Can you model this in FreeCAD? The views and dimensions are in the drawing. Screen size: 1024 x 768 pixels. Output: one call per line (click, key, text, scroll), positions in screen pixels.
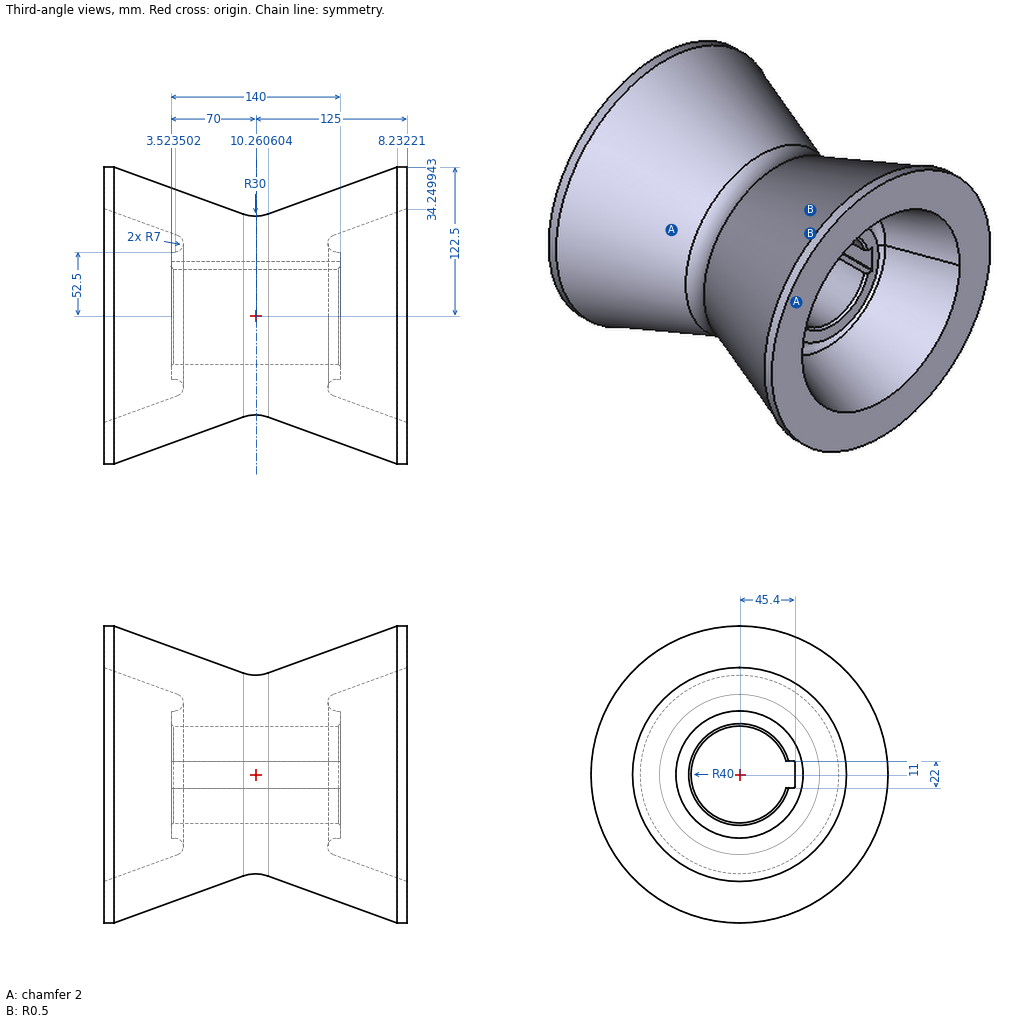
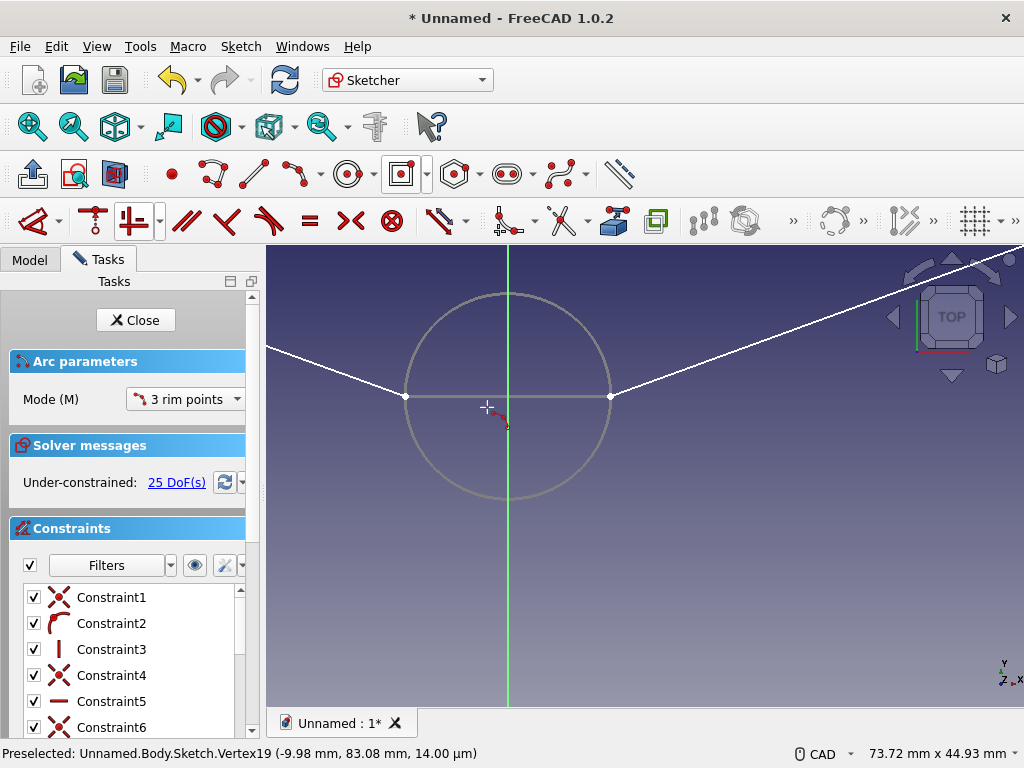
click(486, 408)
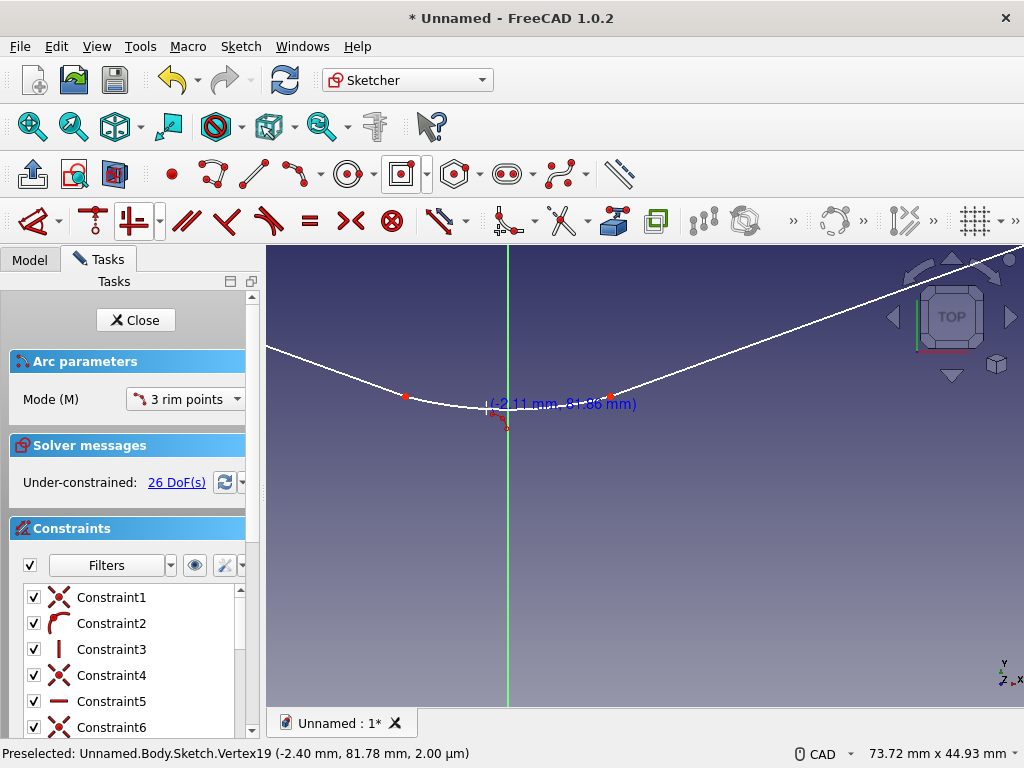
scroll(590, 447, down, 9)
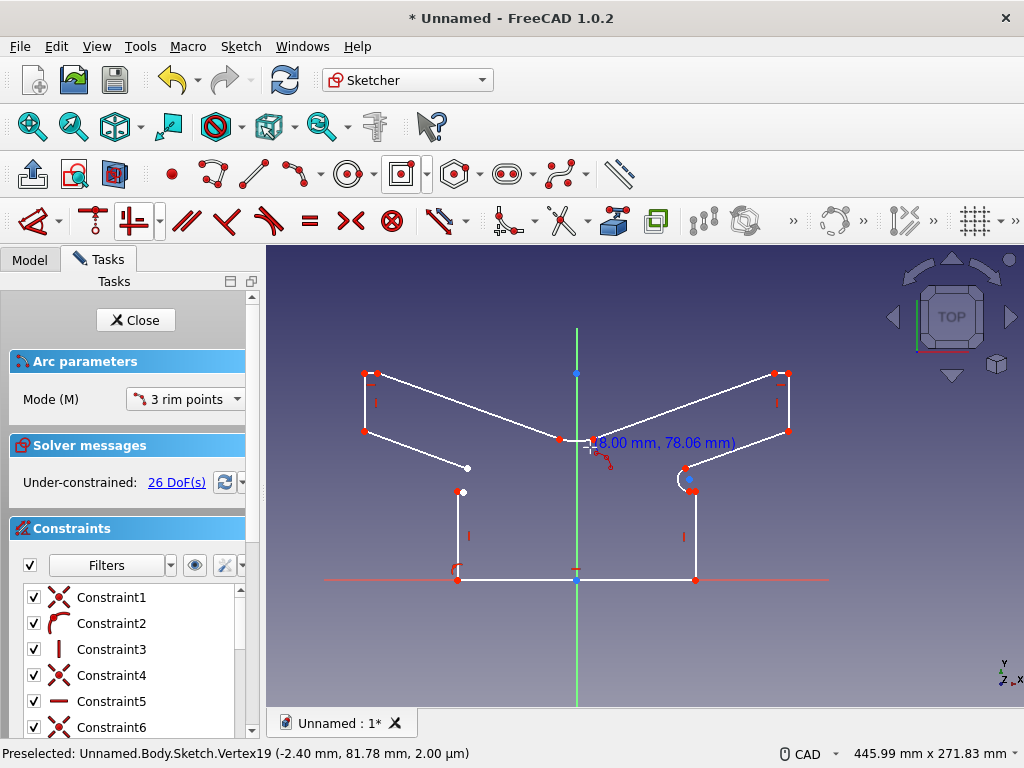
click(468, 469)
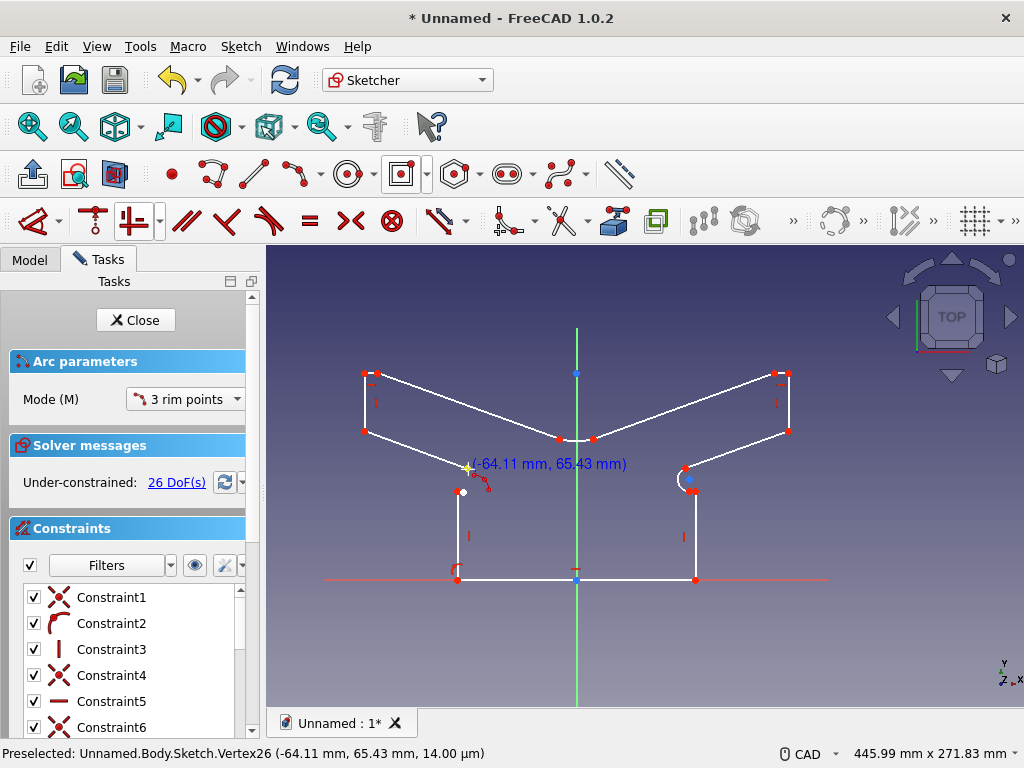
scroll(464, 491, up, 9)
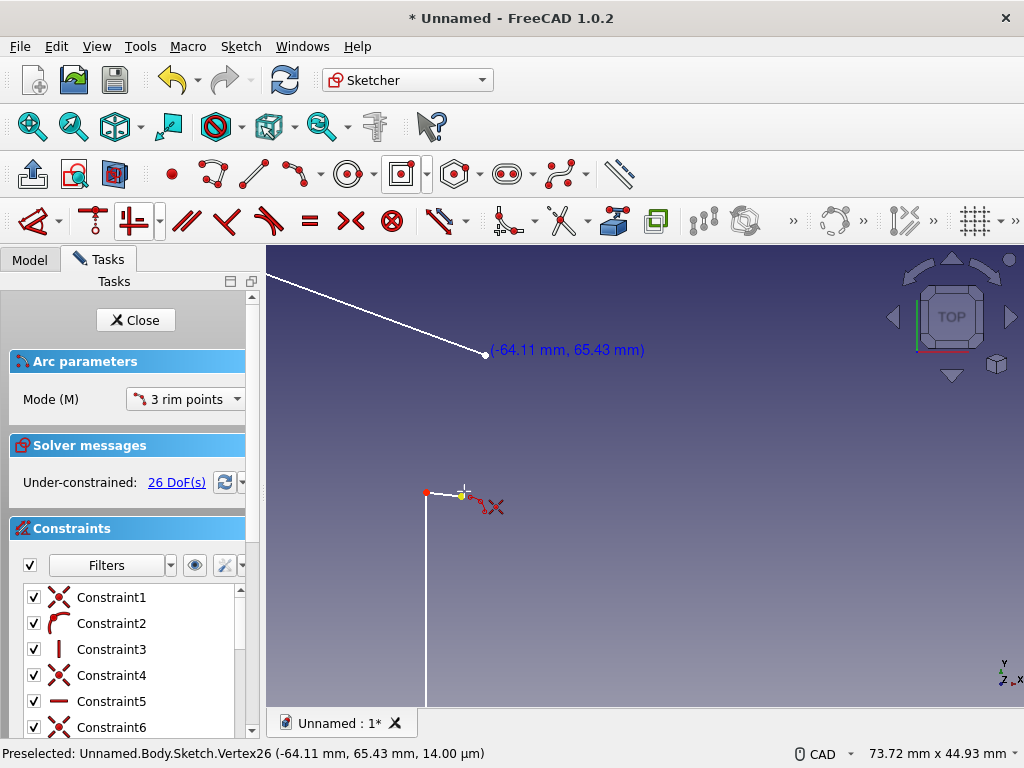
click(461, 497)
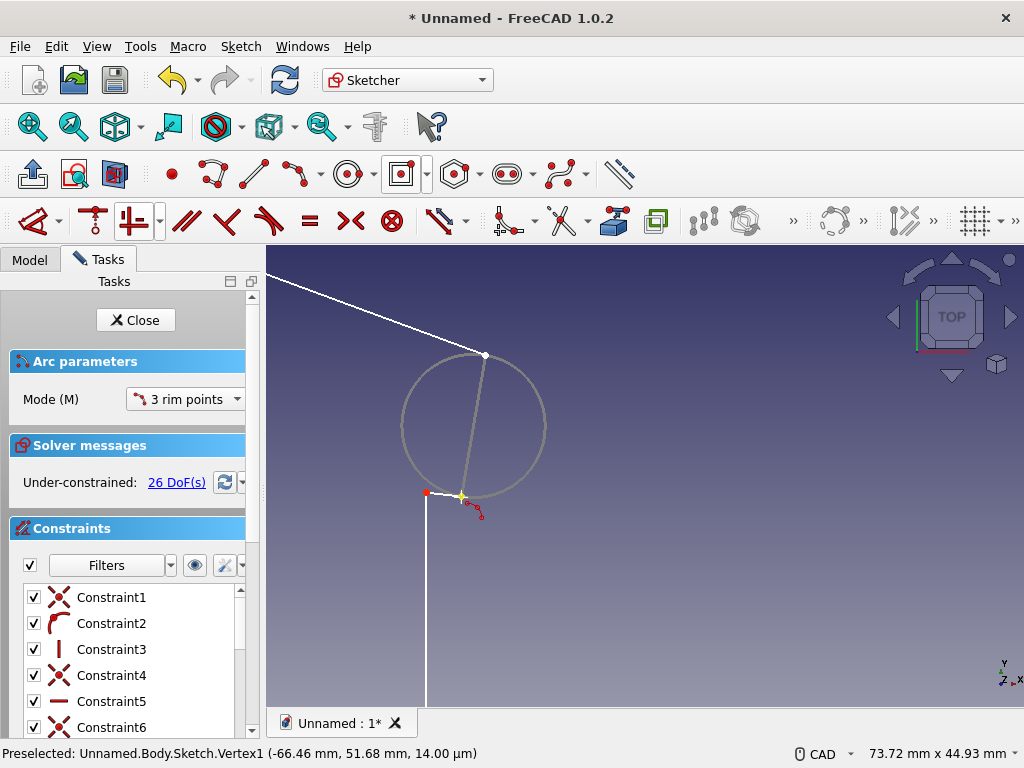
scroll(464, 491, down, 9)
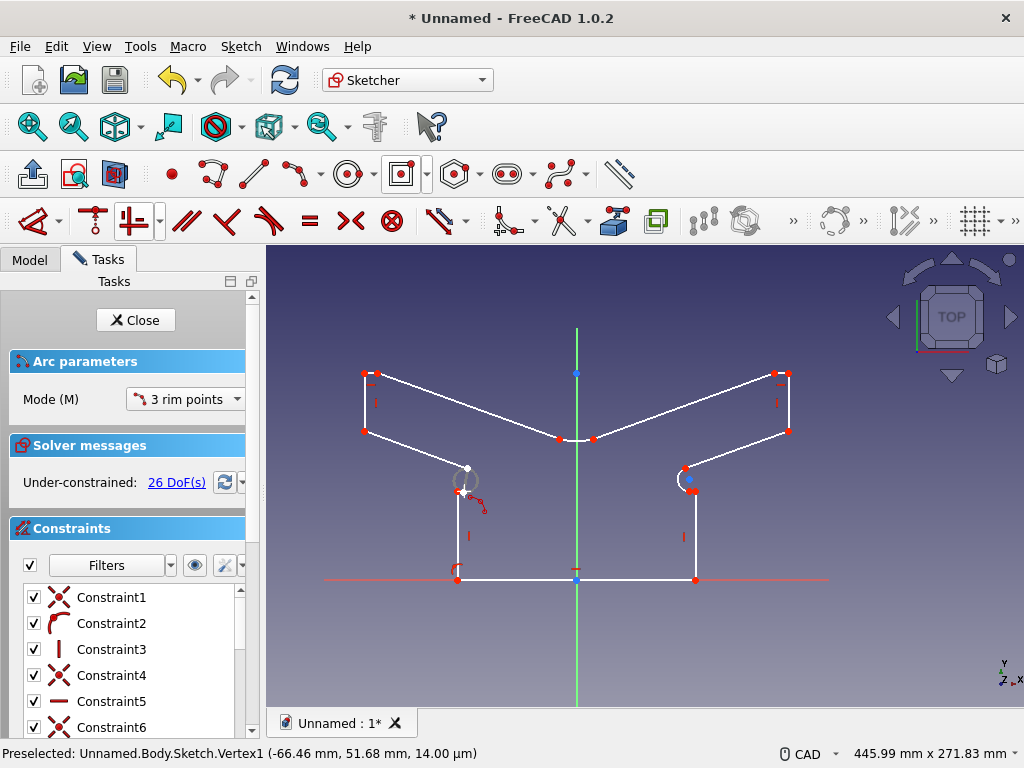
scroll(475, 481, up, 3)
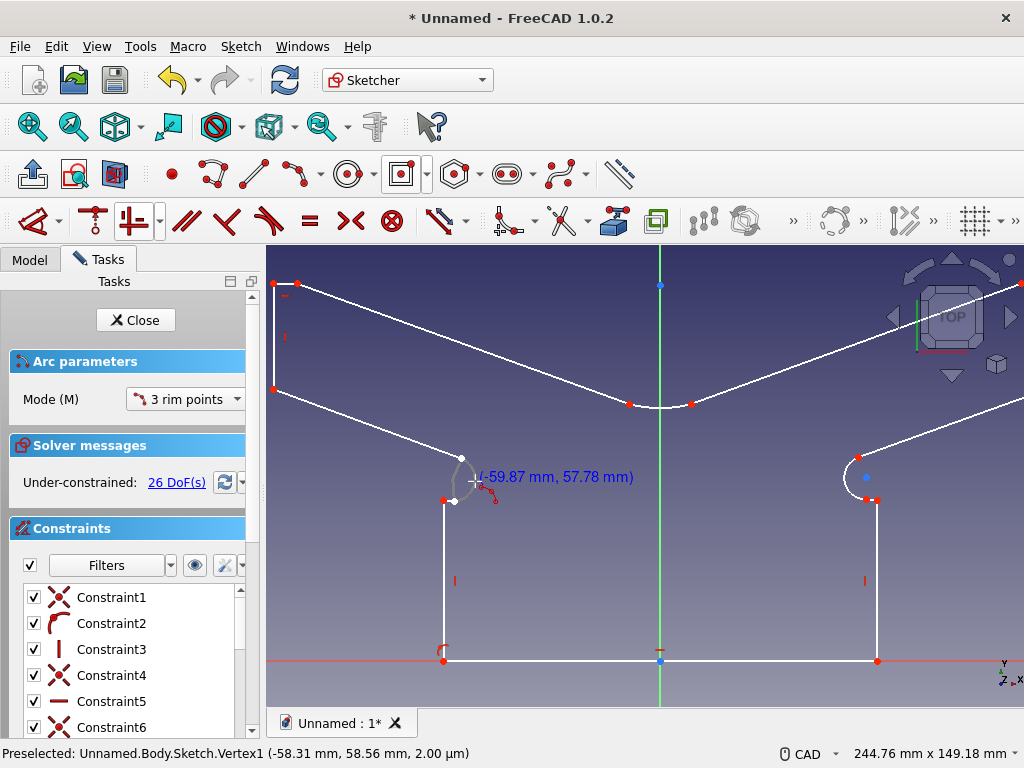
click(476, 481)
key(Escape)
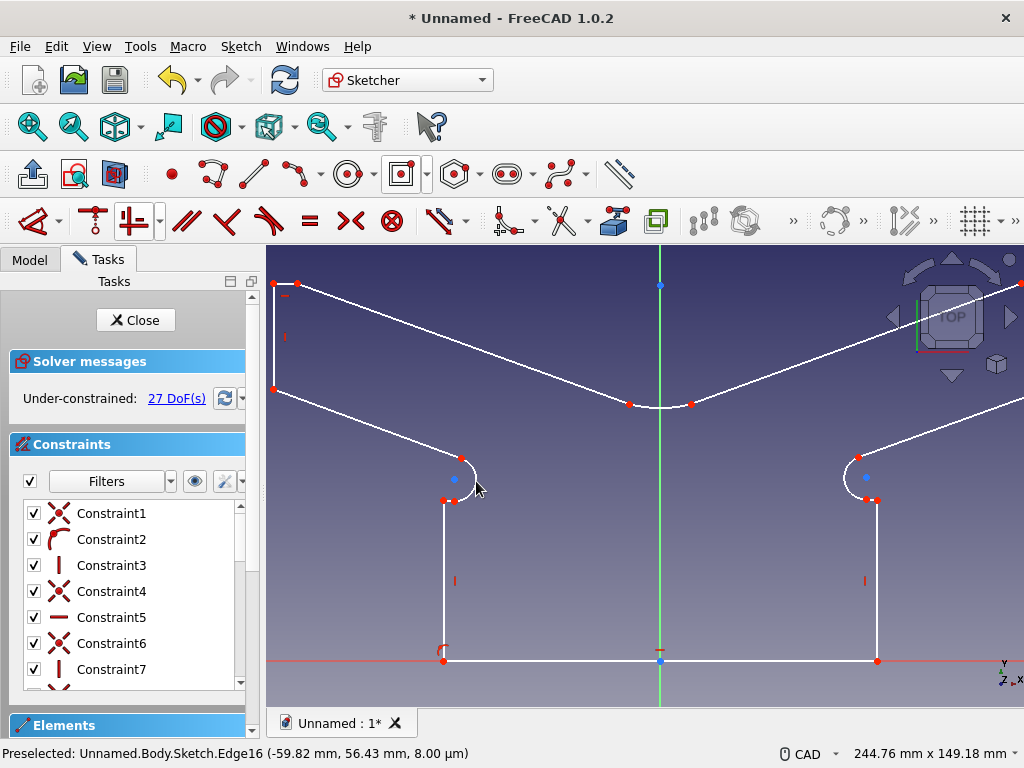
scroll(449, 501, up, 5)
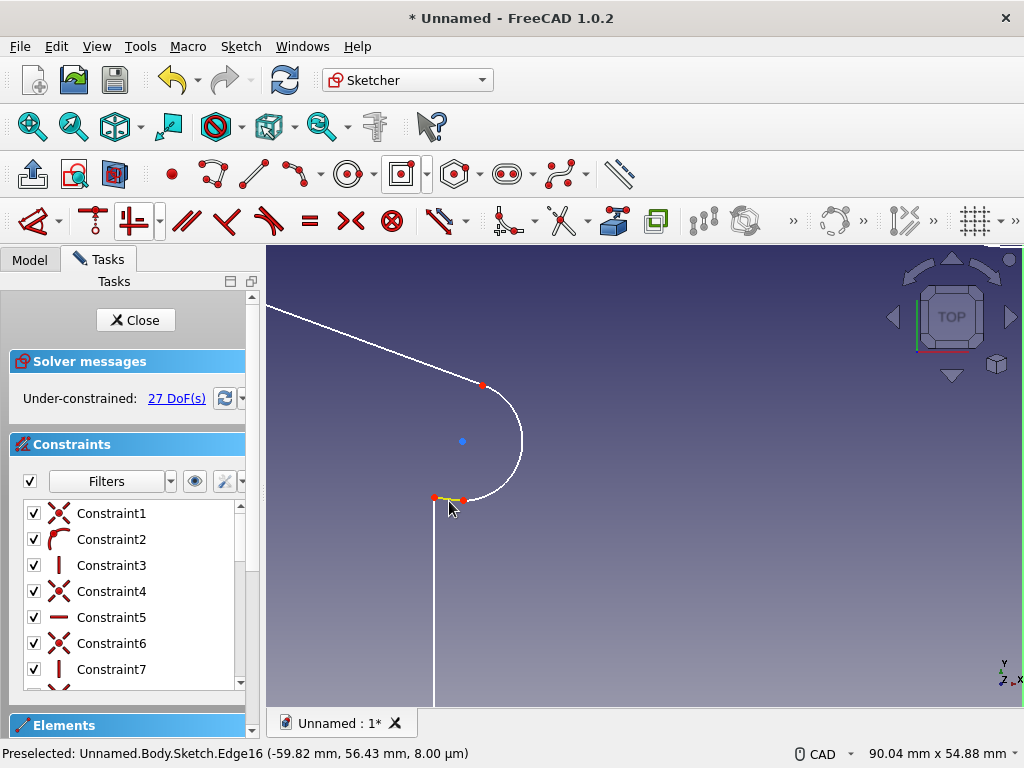
click(449, 499)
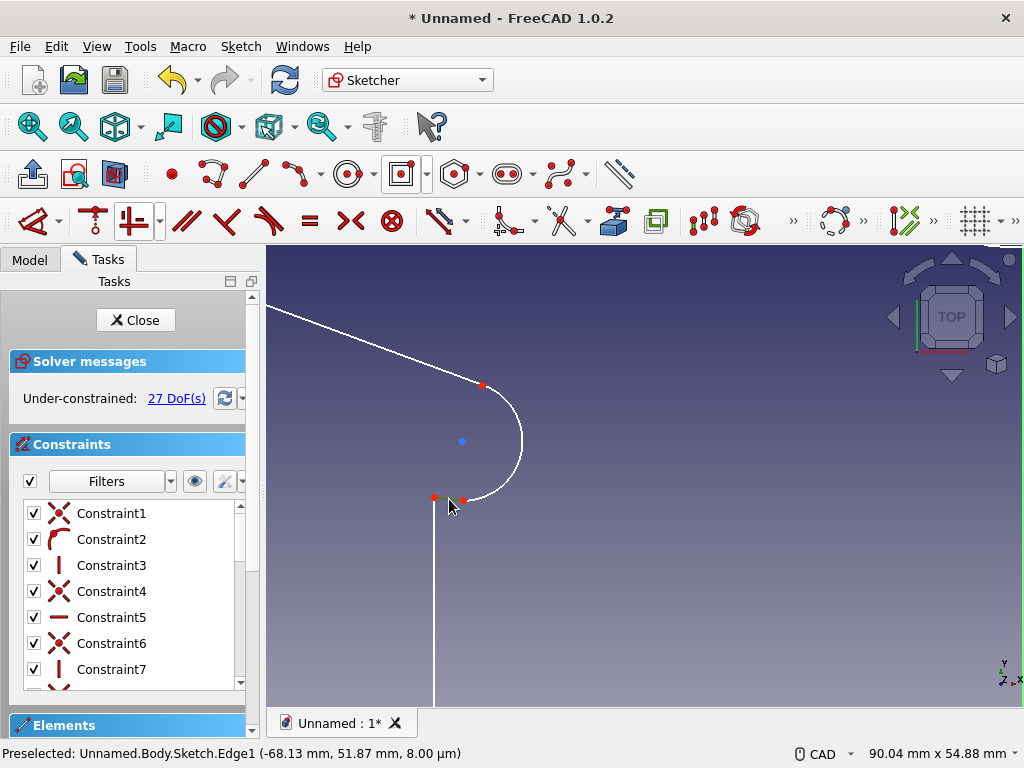
scroll(464, 490, down, 8)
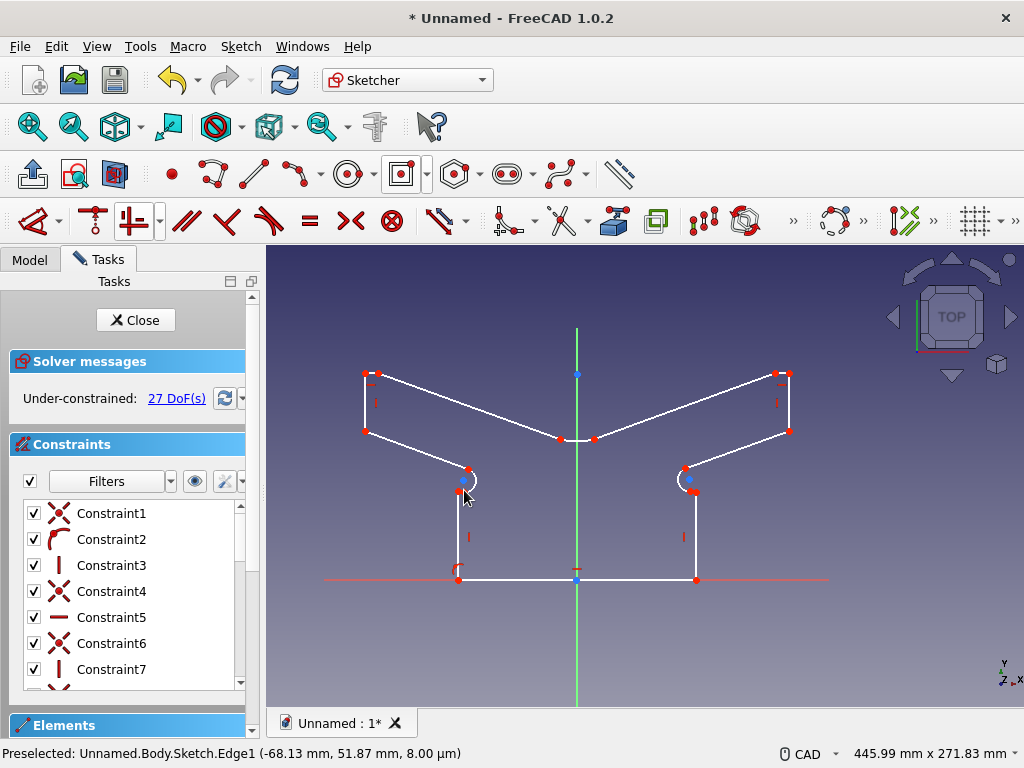
scroll(473, 489, up, 2)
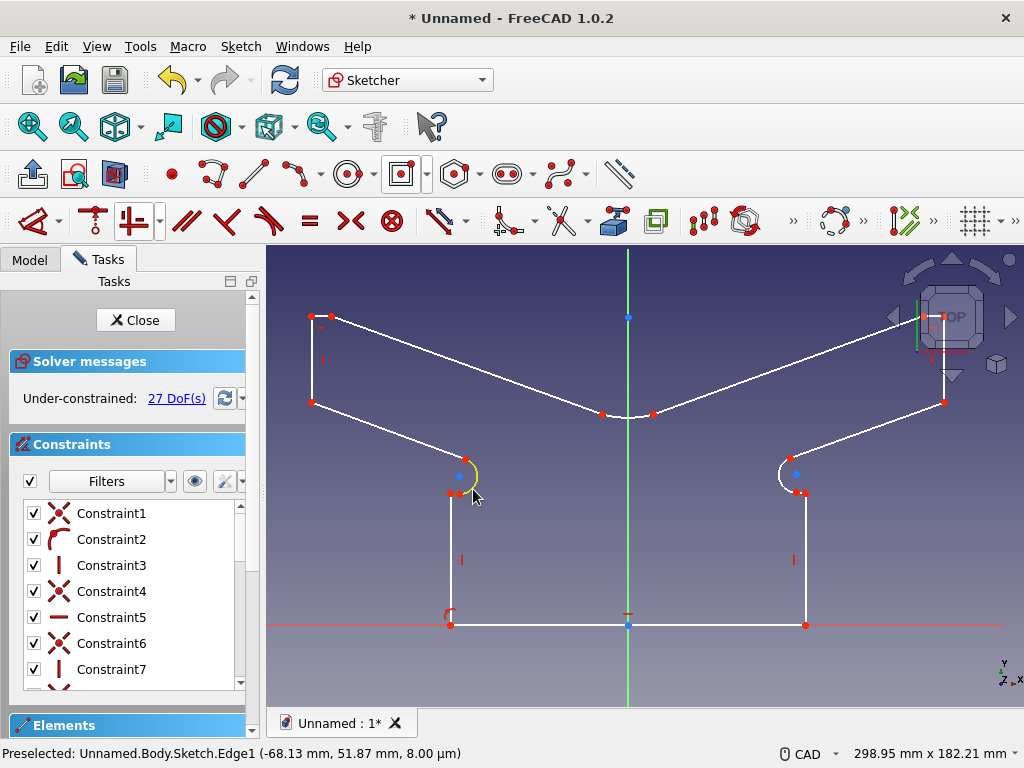
click(473, 488)